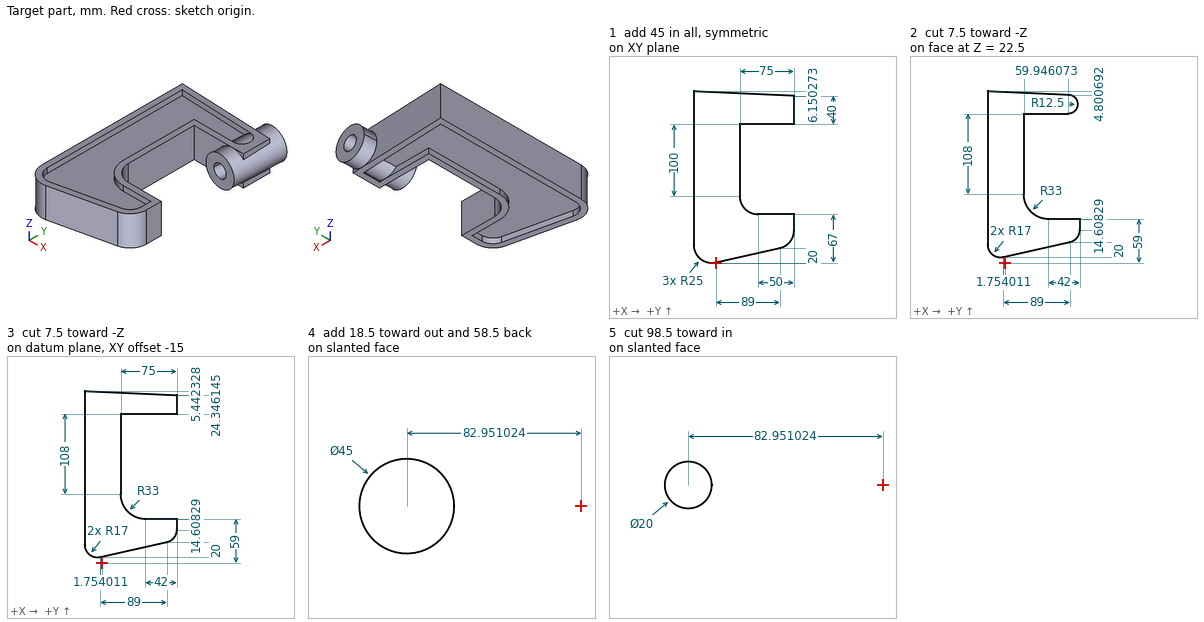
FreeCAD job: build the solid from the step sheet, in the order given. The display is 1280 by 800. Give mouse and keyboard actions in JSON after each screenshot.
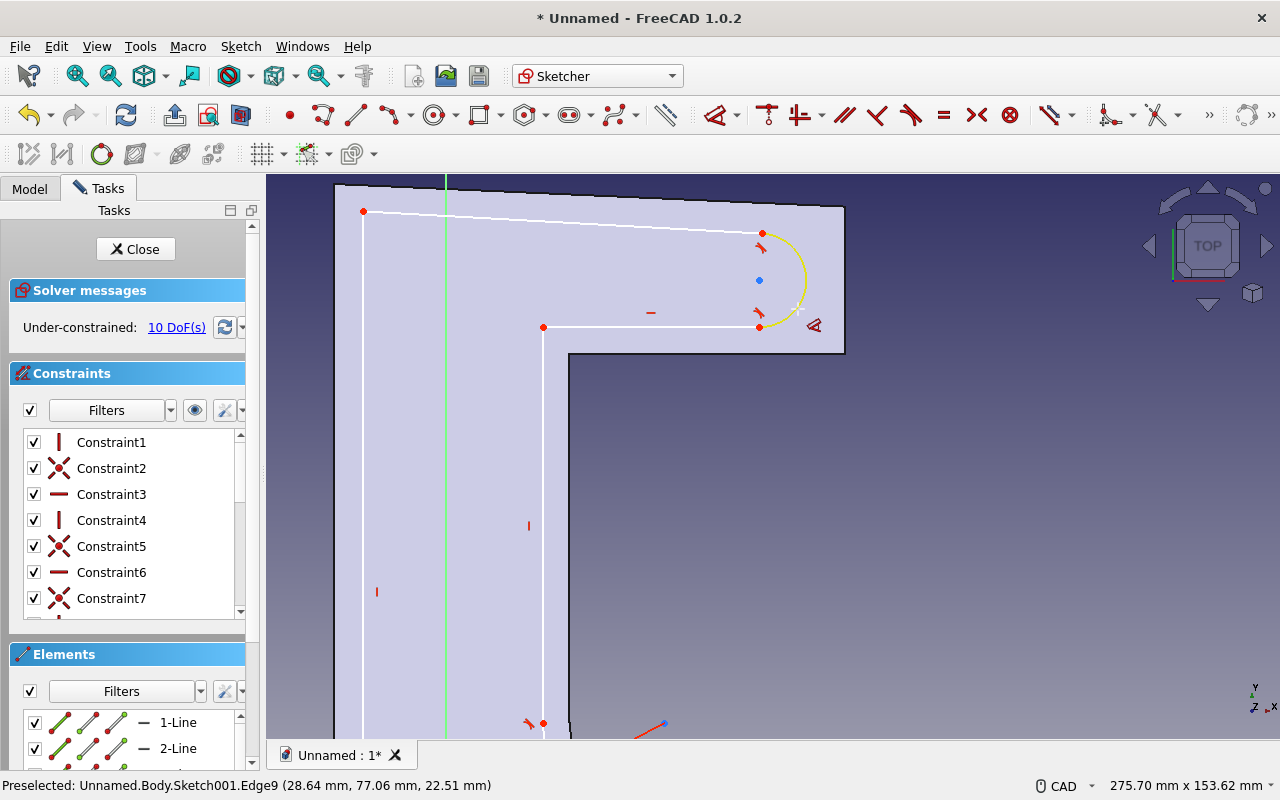
{"action": "left_click", "coordinate": [797, 308]}
{"action": "left_click", "coordinate": [823, 327]}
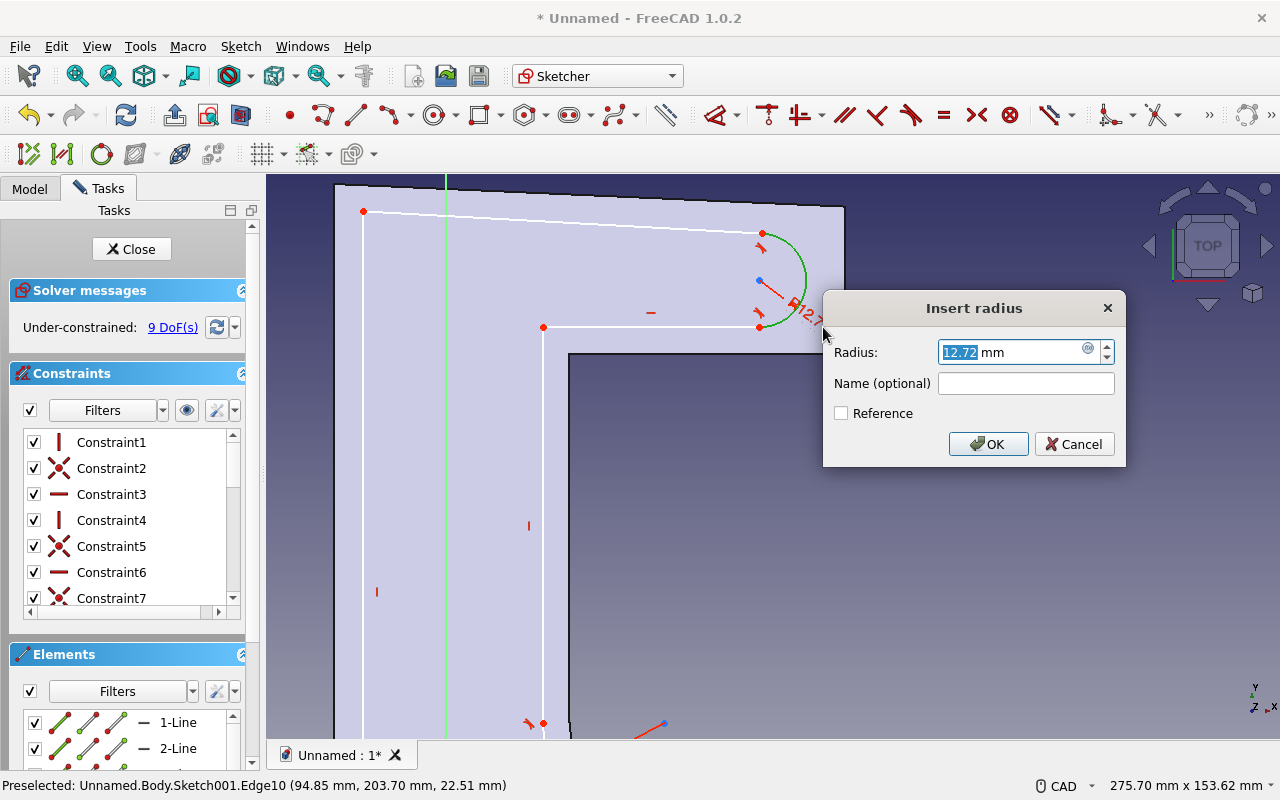
{"action": "type", "text": "12.5"}
{"action": "key", "text": "Return"}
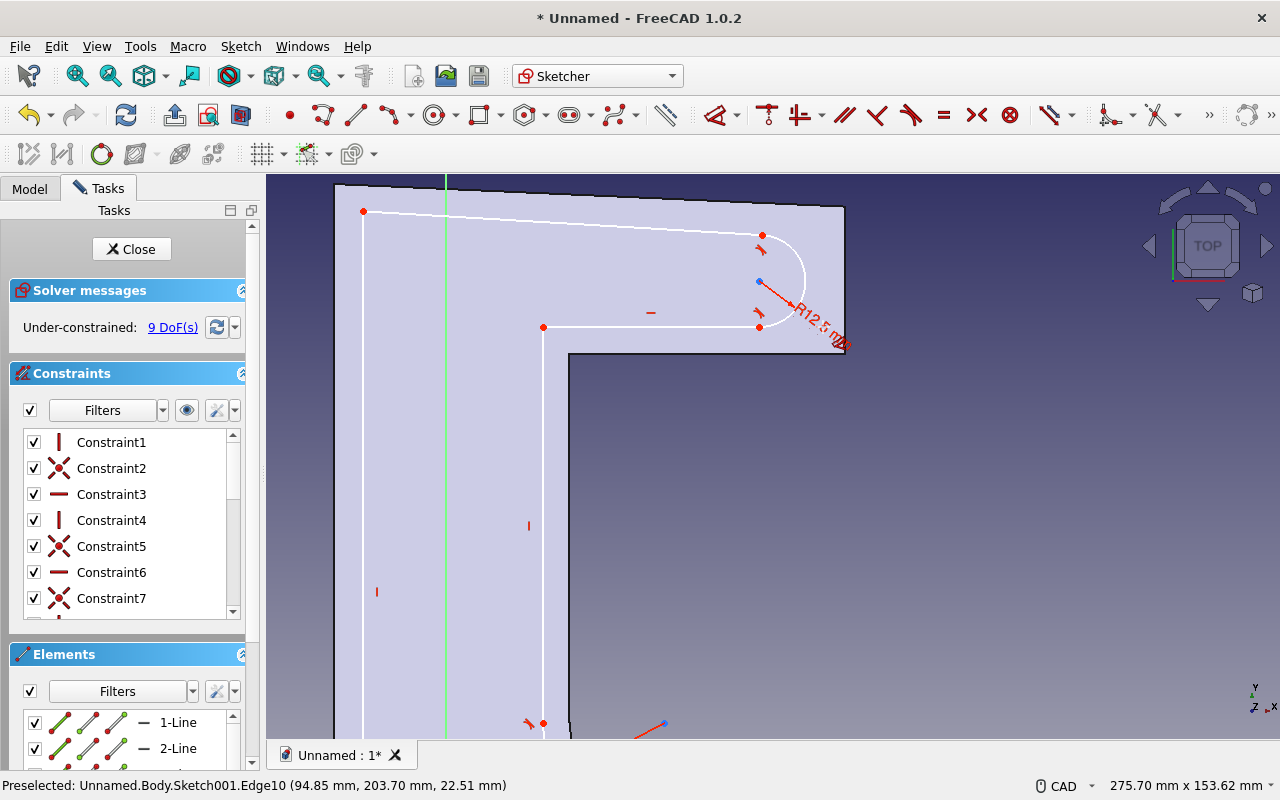
{"action": "scroll", "coordinate": [798, 309], "scroll_direction": "down", "scroll_amount": 4}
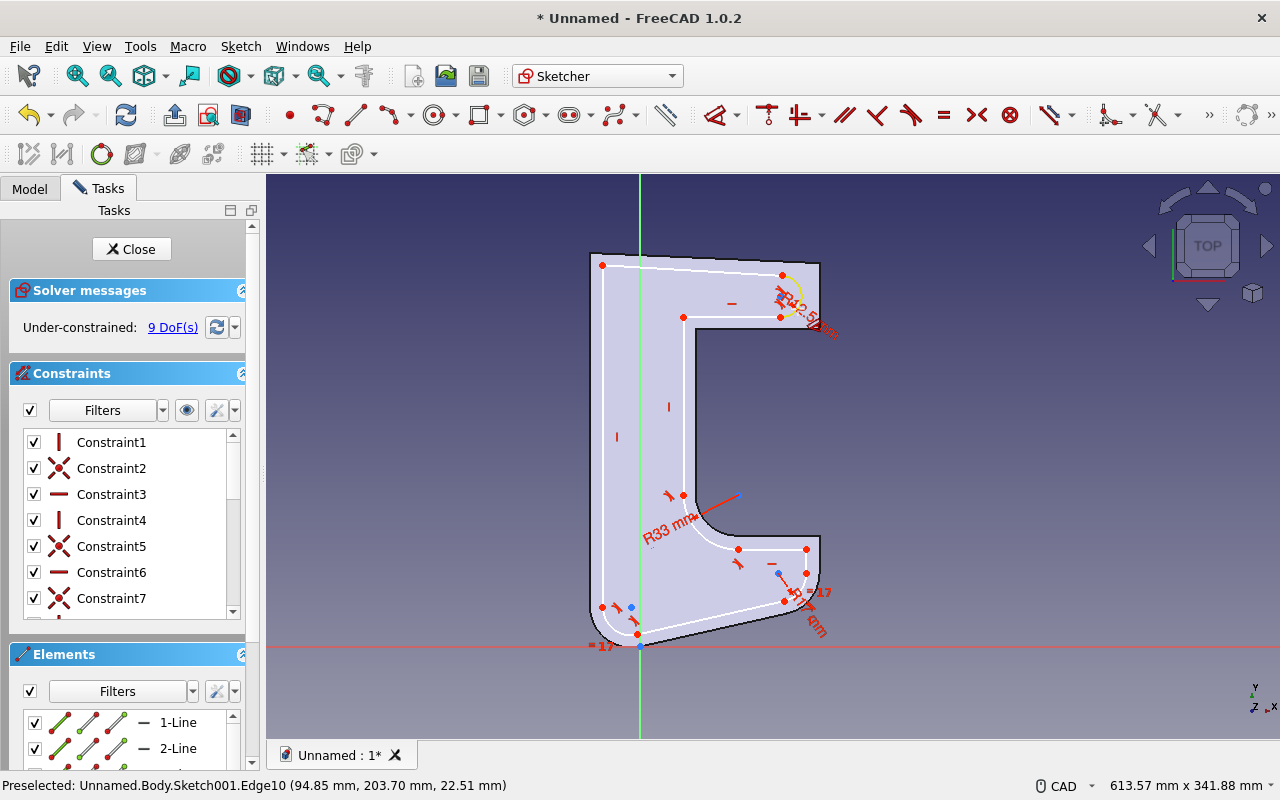
{"action": "left_click", "coordinate": [786, 550]}
{"action": "left_click", "coordinate": [772, 584]}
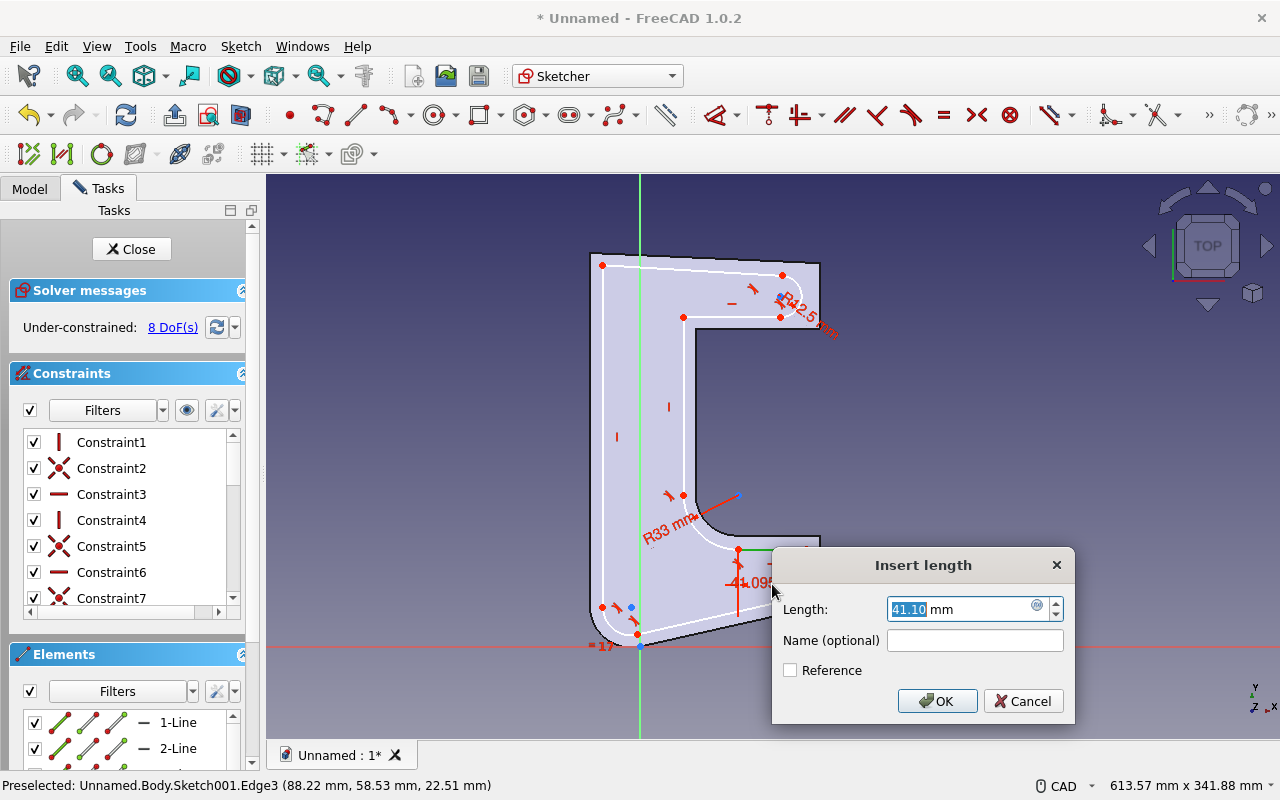
{"action": "type", "text": "42"}
{"action": "key", "text": "Return"}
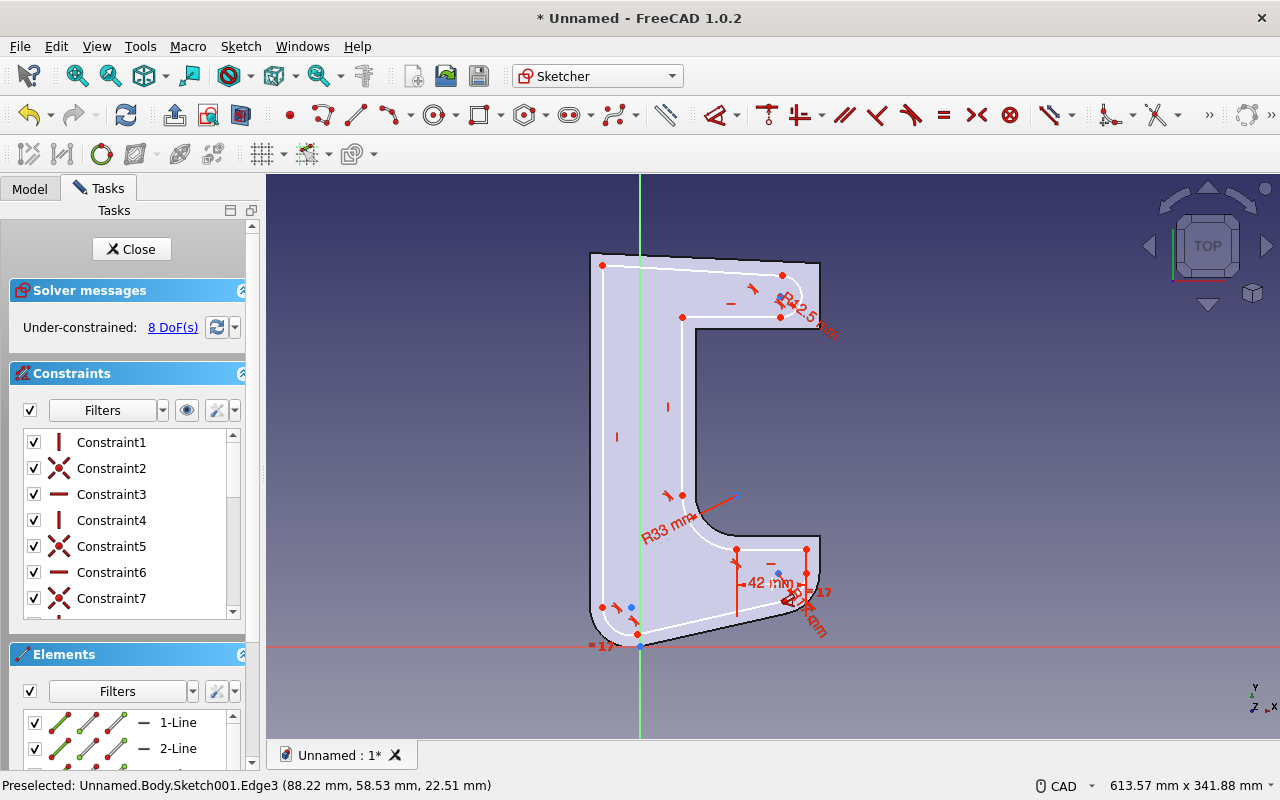
{"action": "left_click", "coordinate": [682, 442]}
{"action": "left_click", "coordinate": [716, 406]}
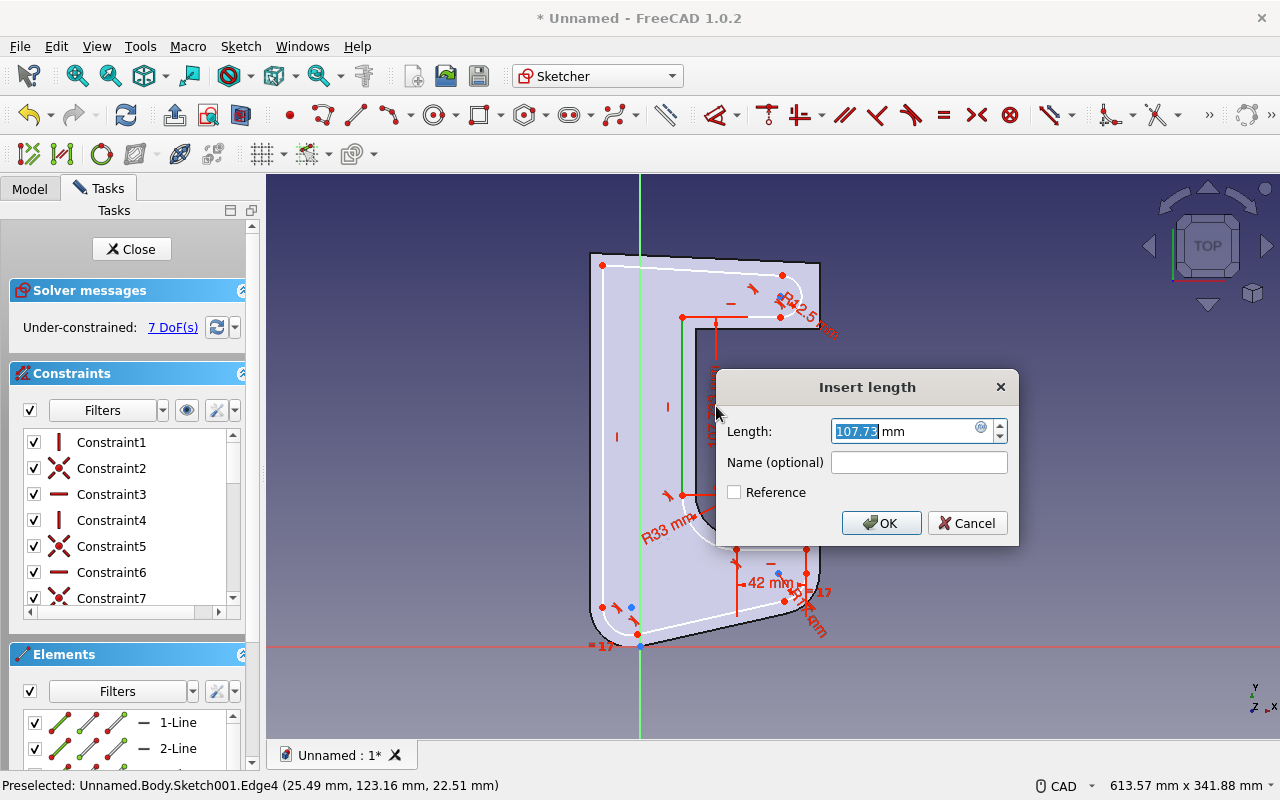
{"action": "type", "text": "108"}
{"action": "key", "text": "Return"}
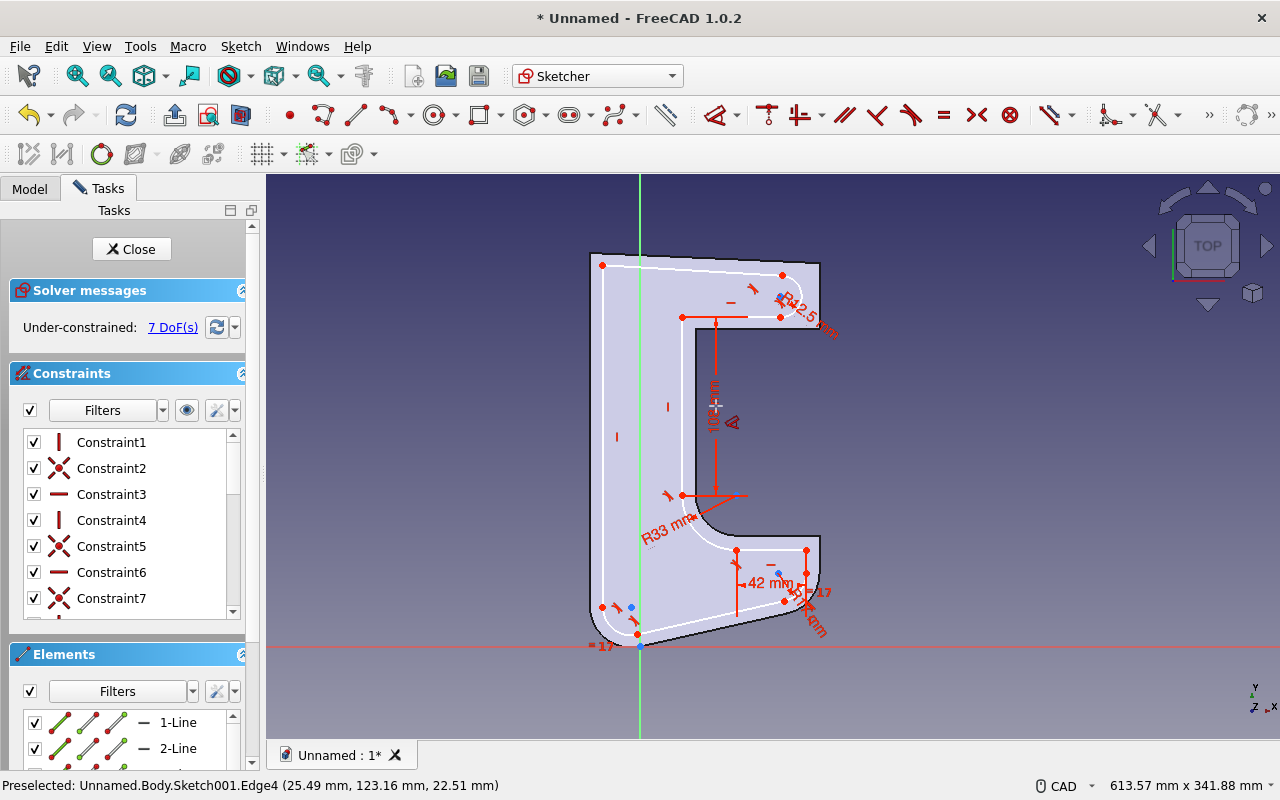
{"action": "left_click", "coordinate": [806, 550]}
{"action": "left_click", "coordinate": [864, 576]}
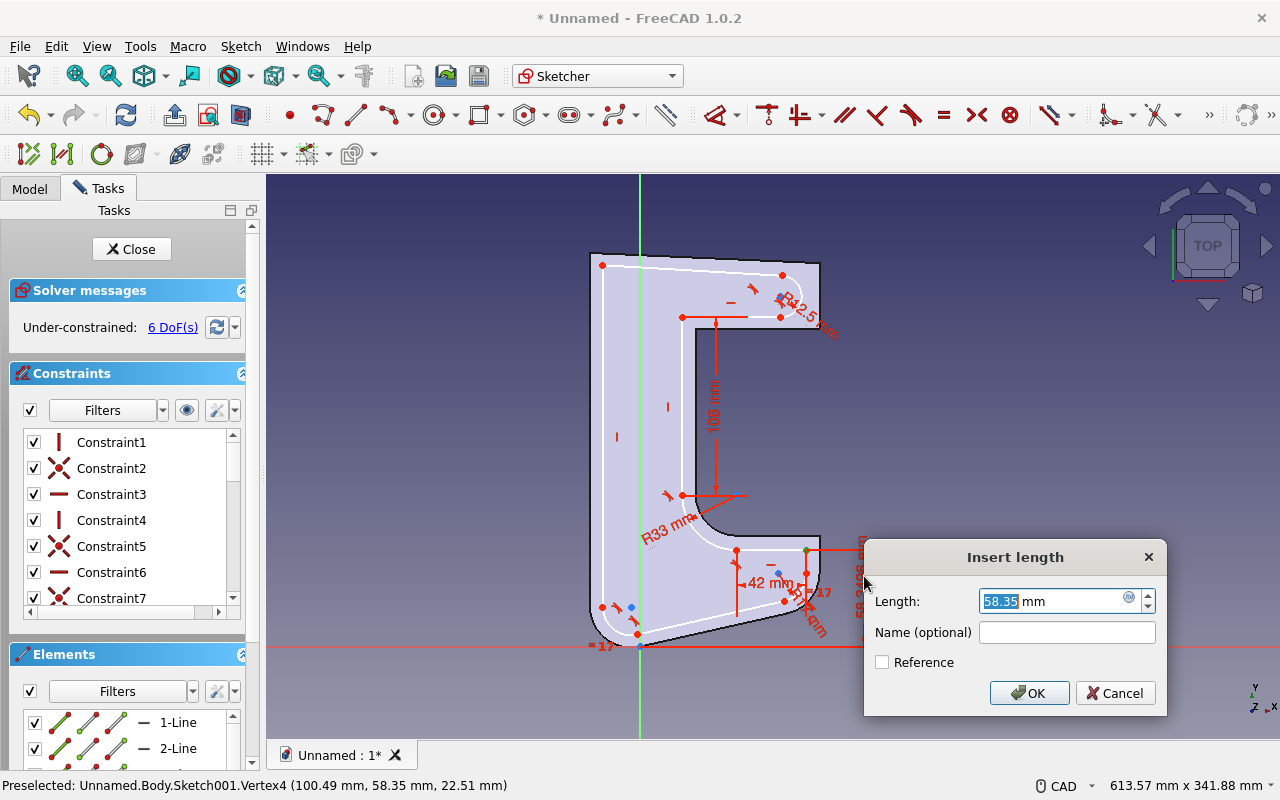
{"action": "type", "text": "59"}
{"action": "key", "text": "Return"}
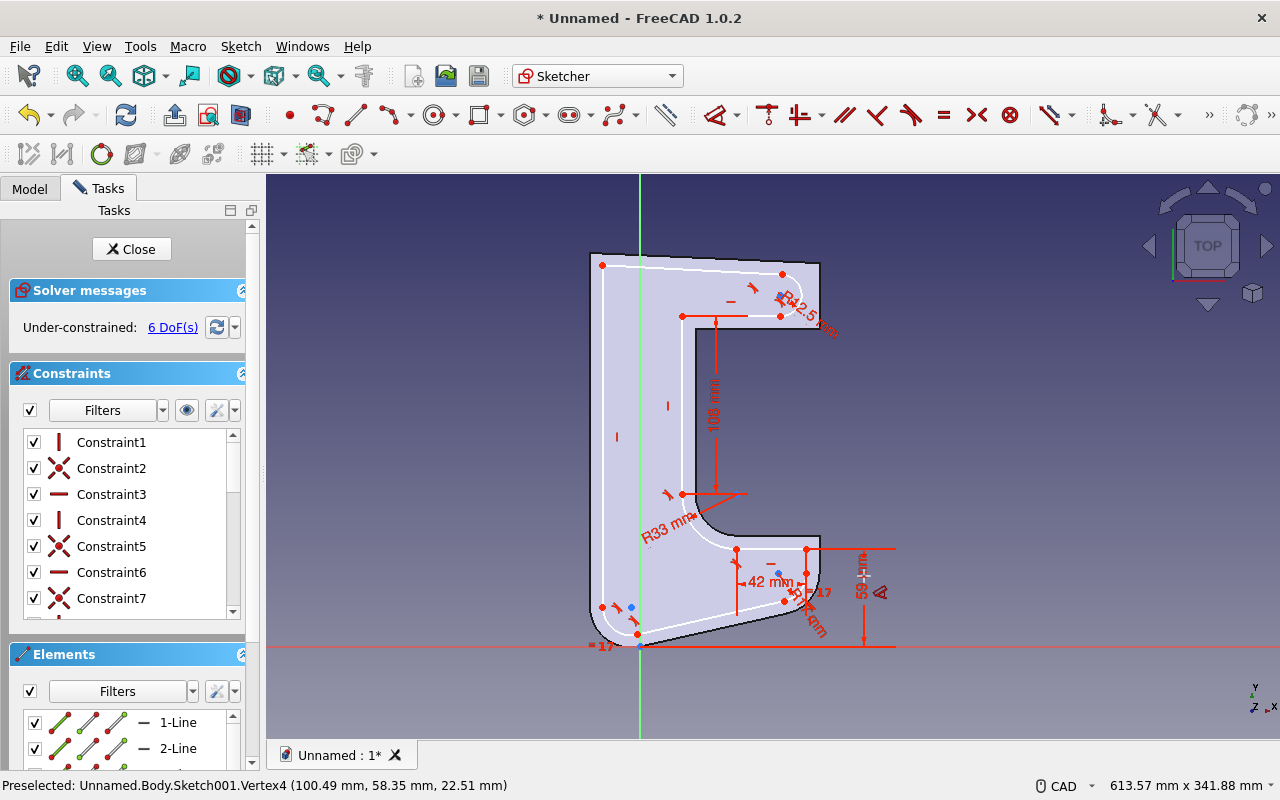
{"action": "left_click", "coordinate": [681, 625]}
{"action": "left_click", "coordinate": [711, 669]}